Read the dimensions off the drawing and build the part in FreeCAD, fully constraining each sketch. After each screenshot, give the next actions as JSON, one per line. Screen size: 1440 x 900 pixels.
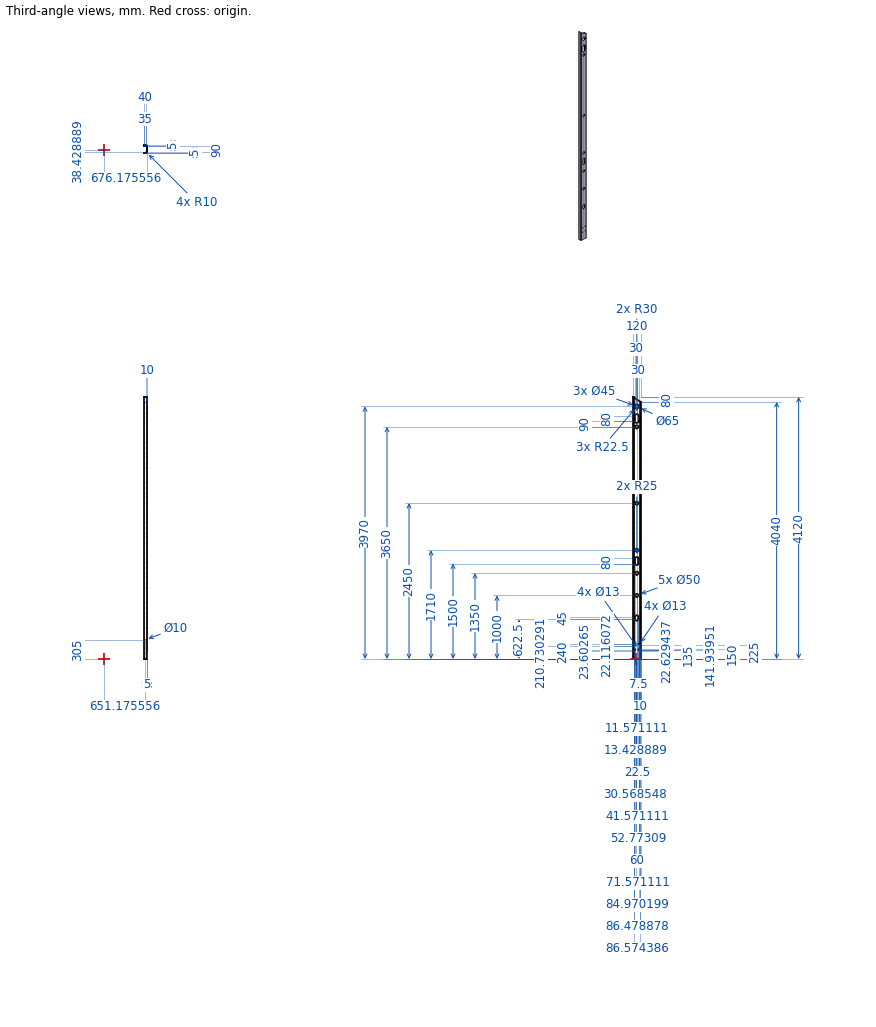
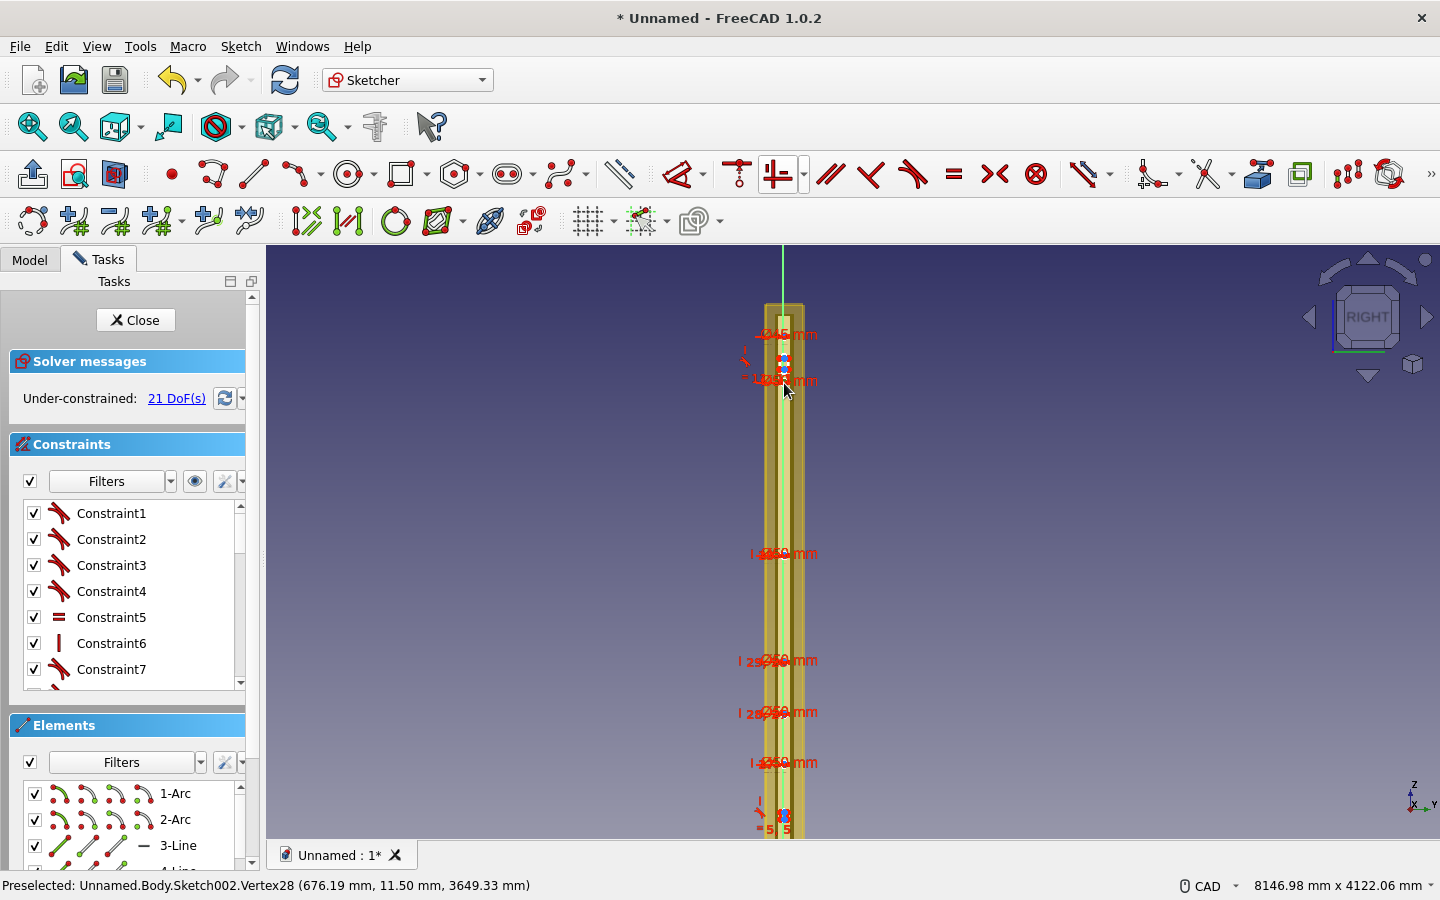
{"action": "left_click", "coordinate": [784, 556]}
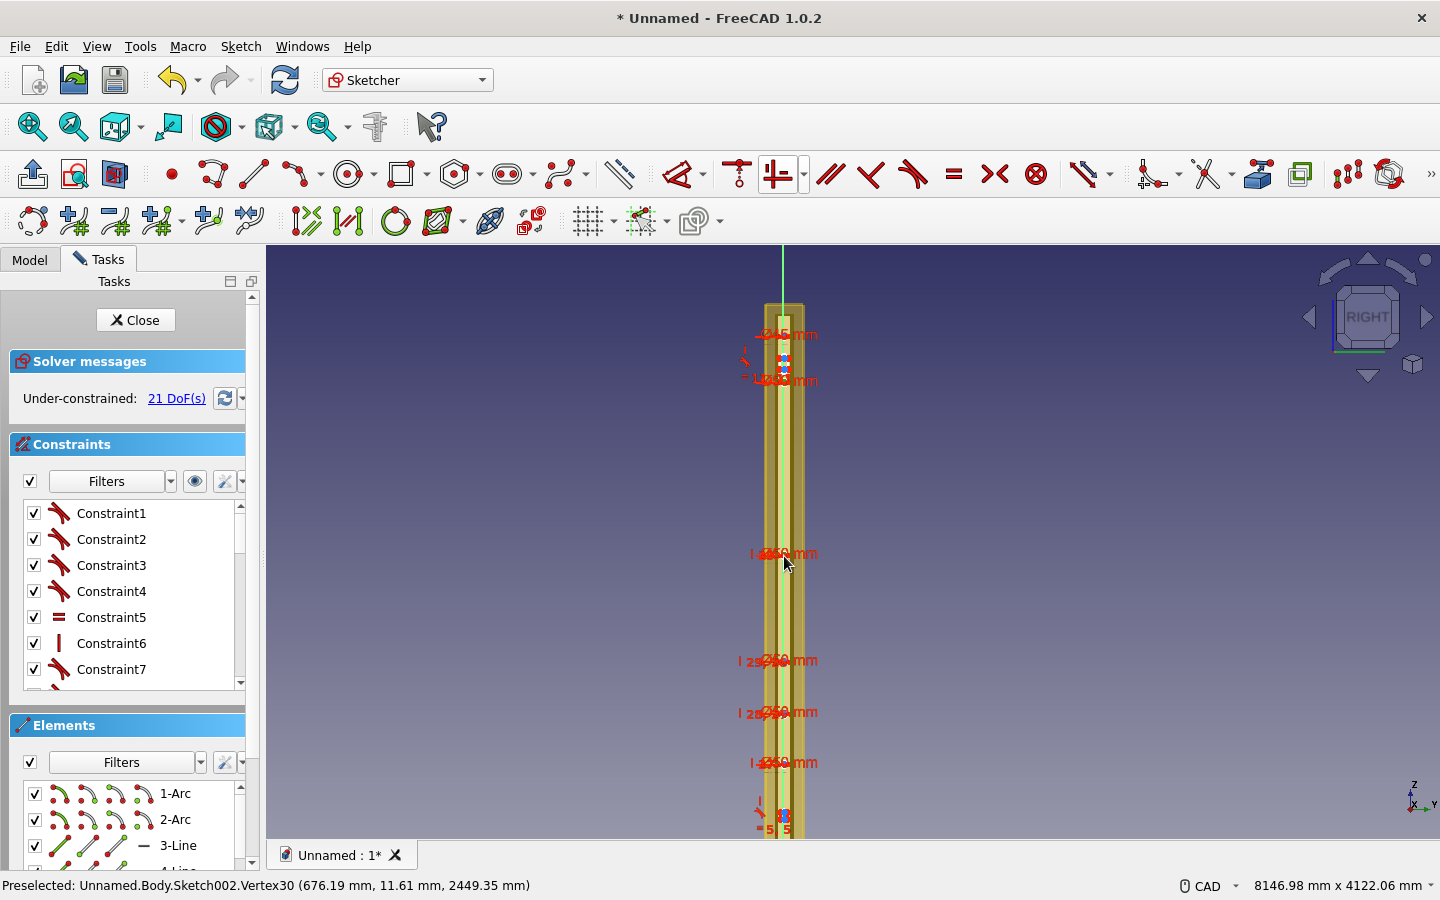
{"action": "key", "text": "v"}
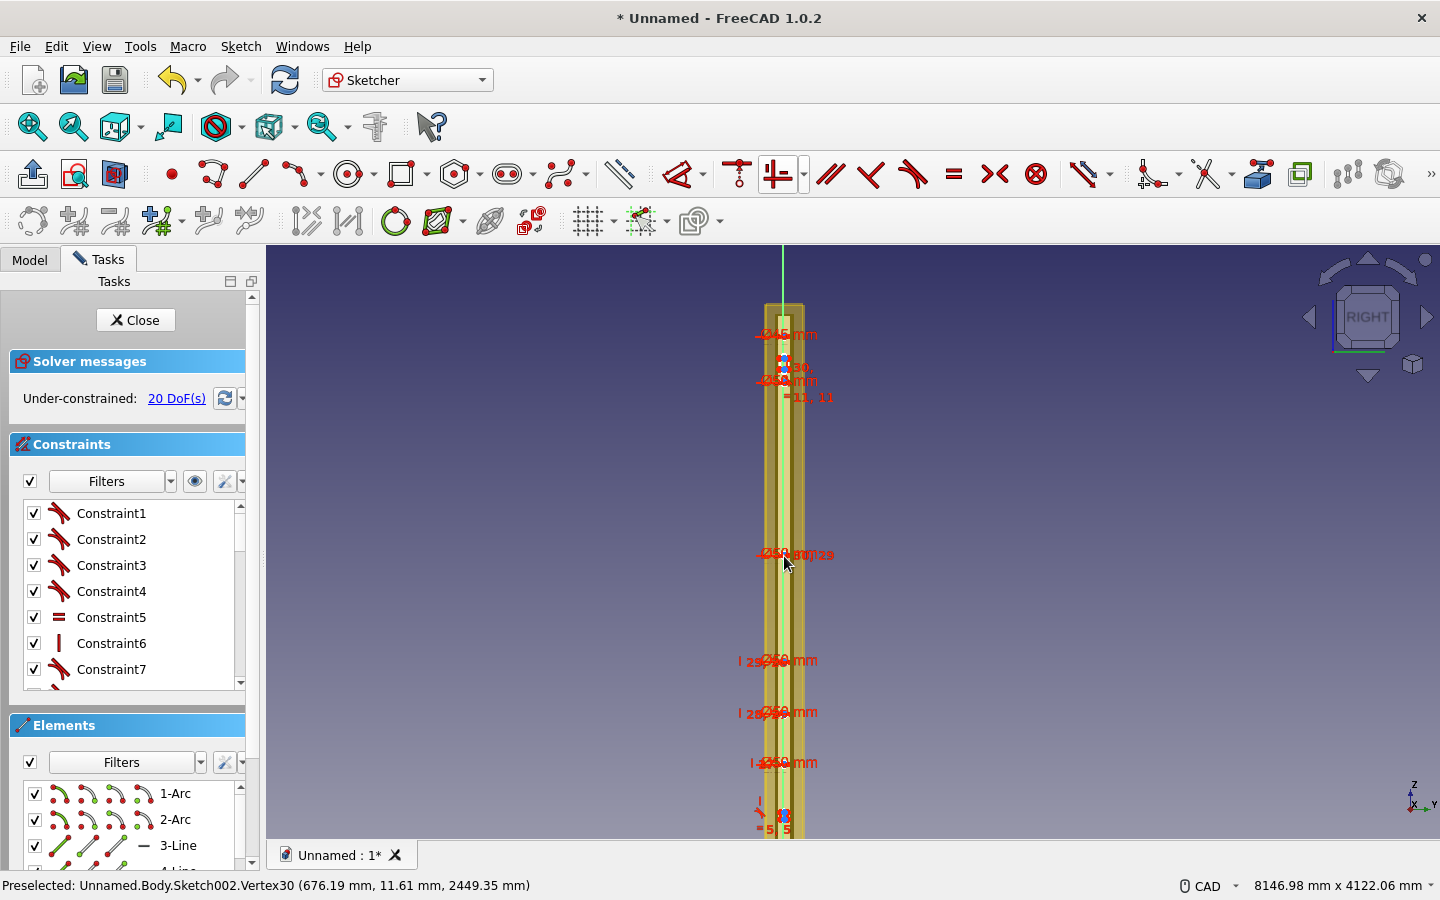
{"action": "key", "text": "d"}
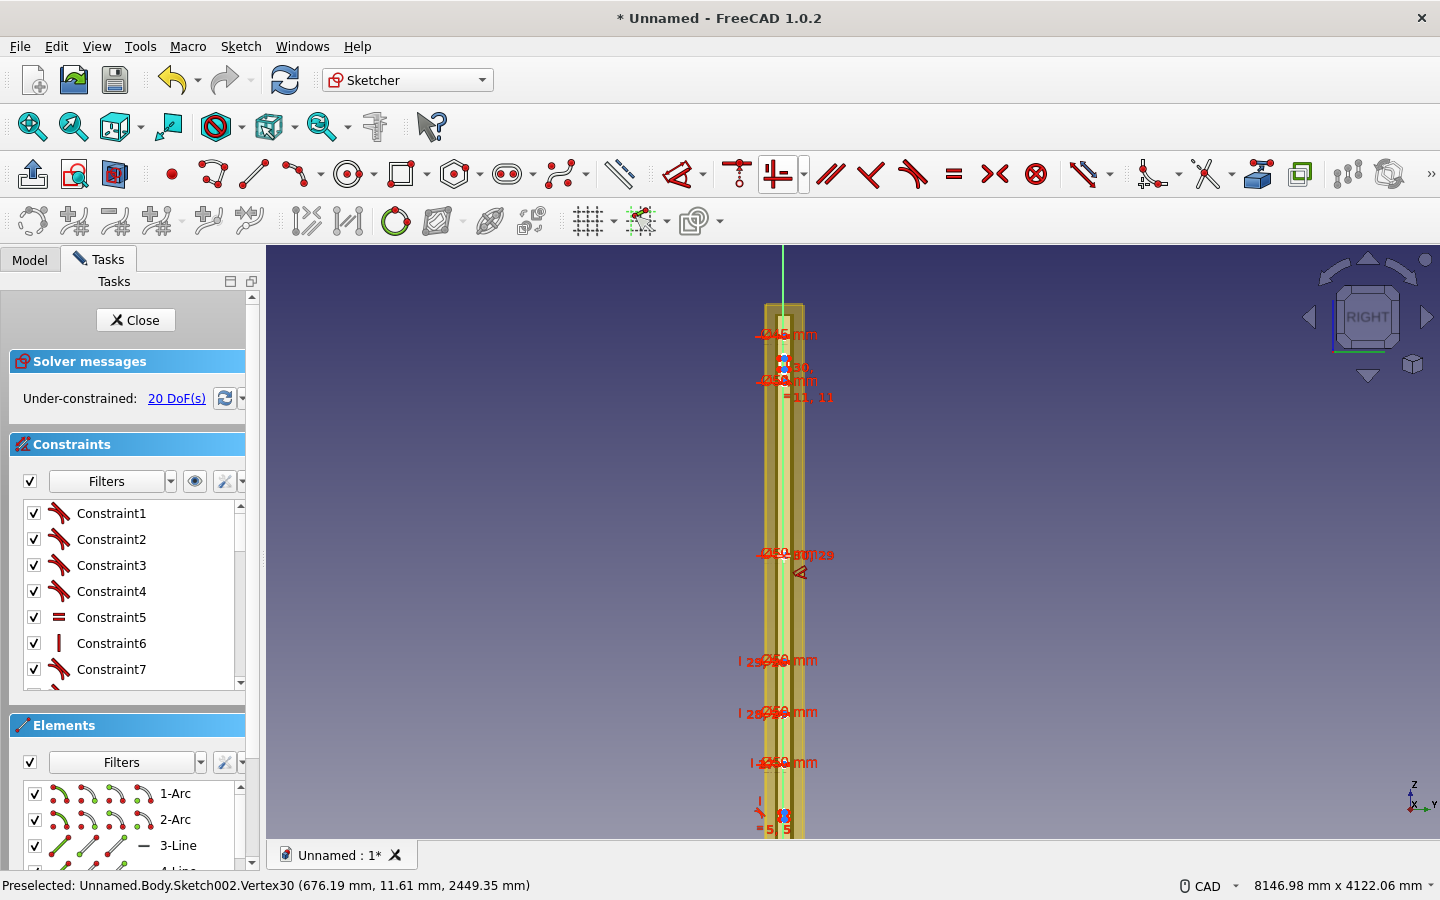
{"action": "scroll", "coordinate": [785, 381], "scroll_direction": "down", "scroll_amount": 2}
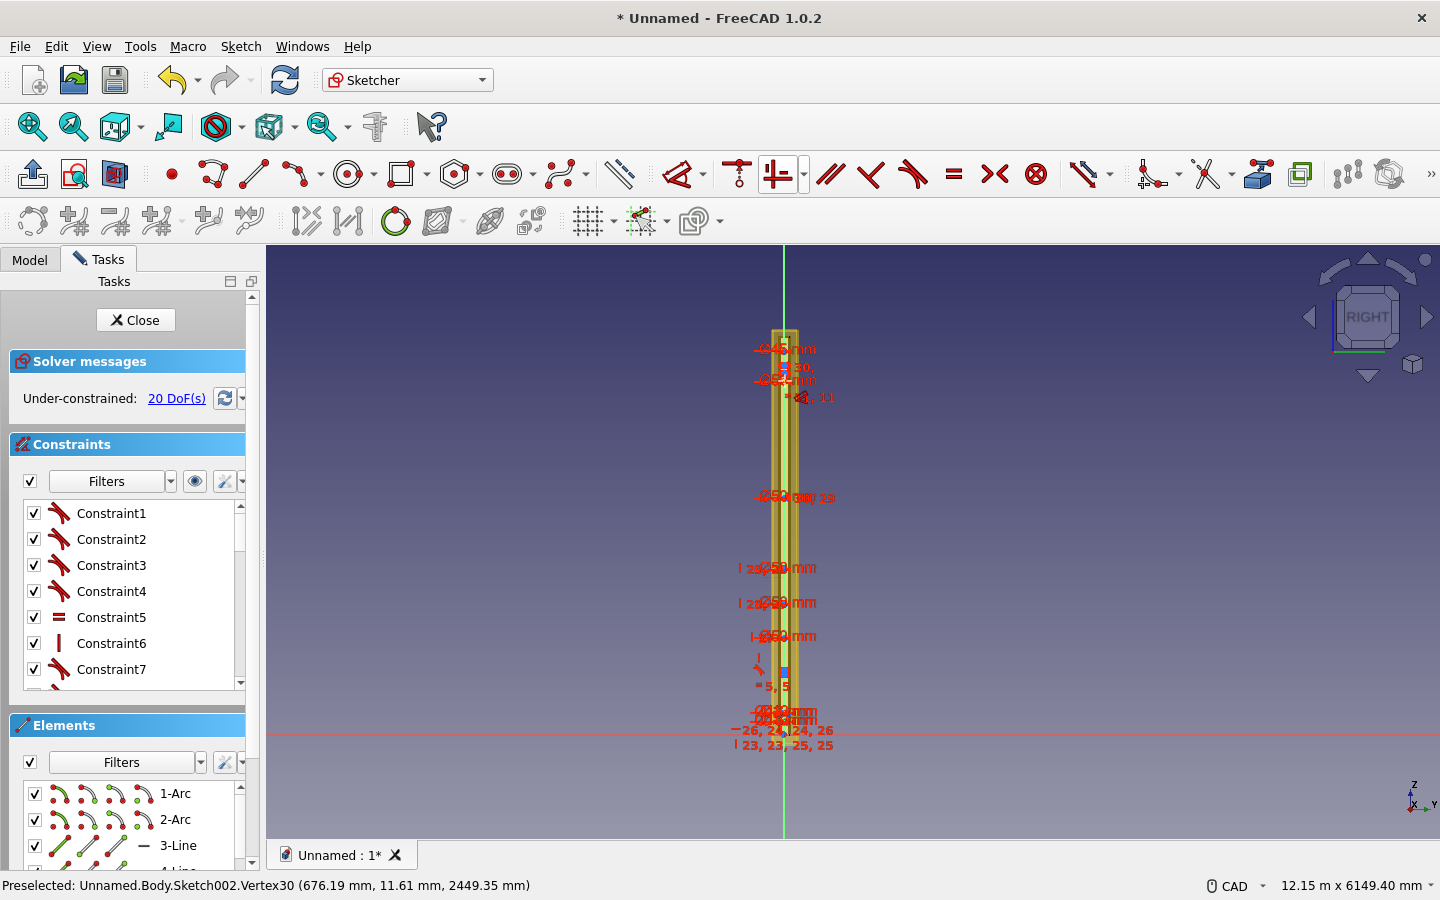
{"action": "scroll", "coordinate": [785, 677], "scroll_direction": "up", "scroll_amount": 15}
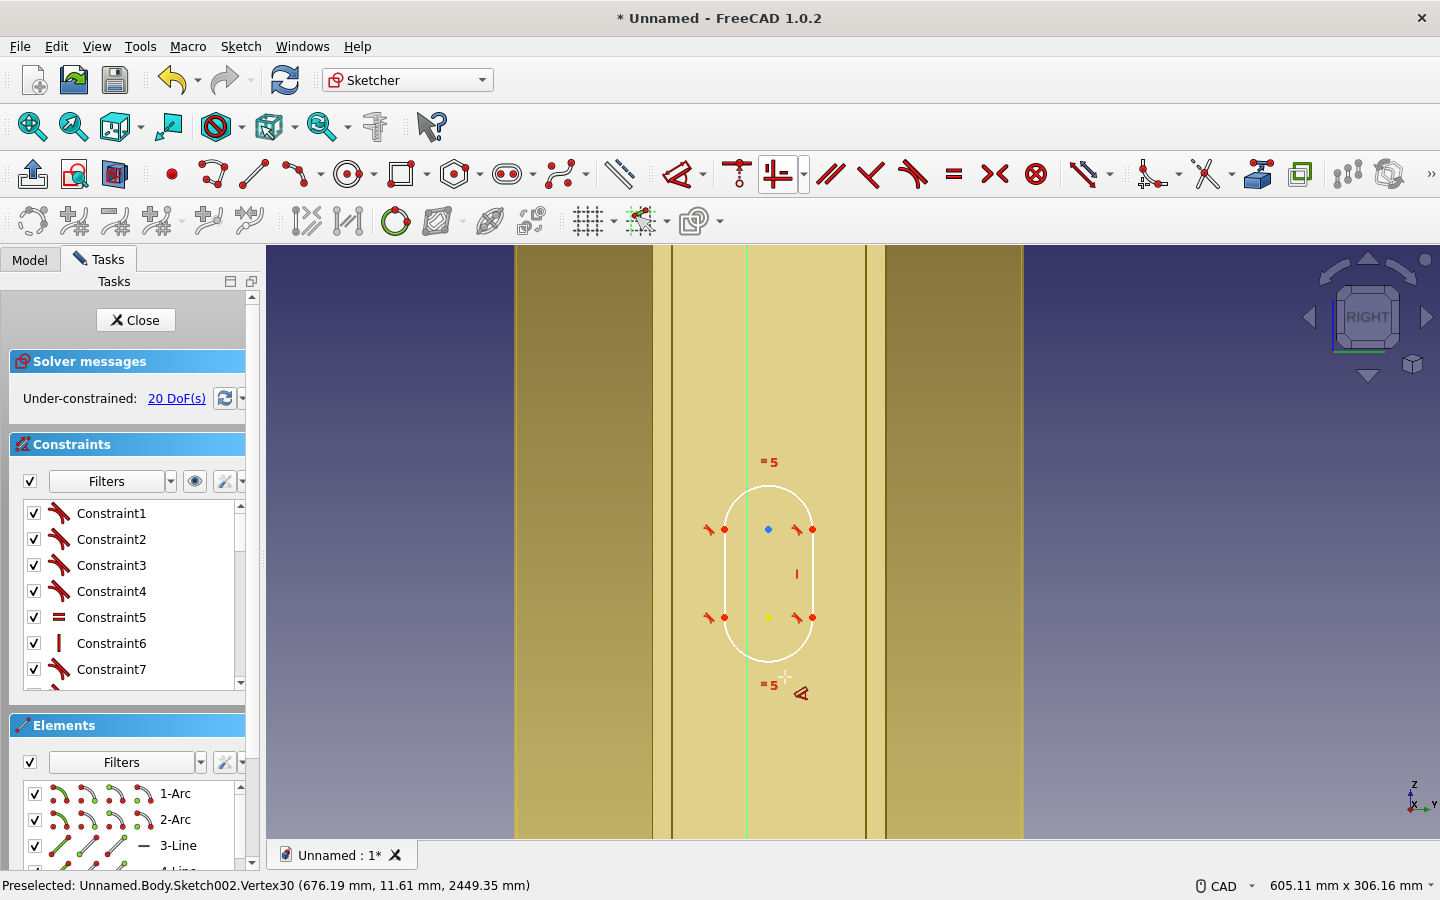
{"action": "left_click", "coordinate": [769, 662]}
{"action": "left_click", "coordinate": [769, 694]}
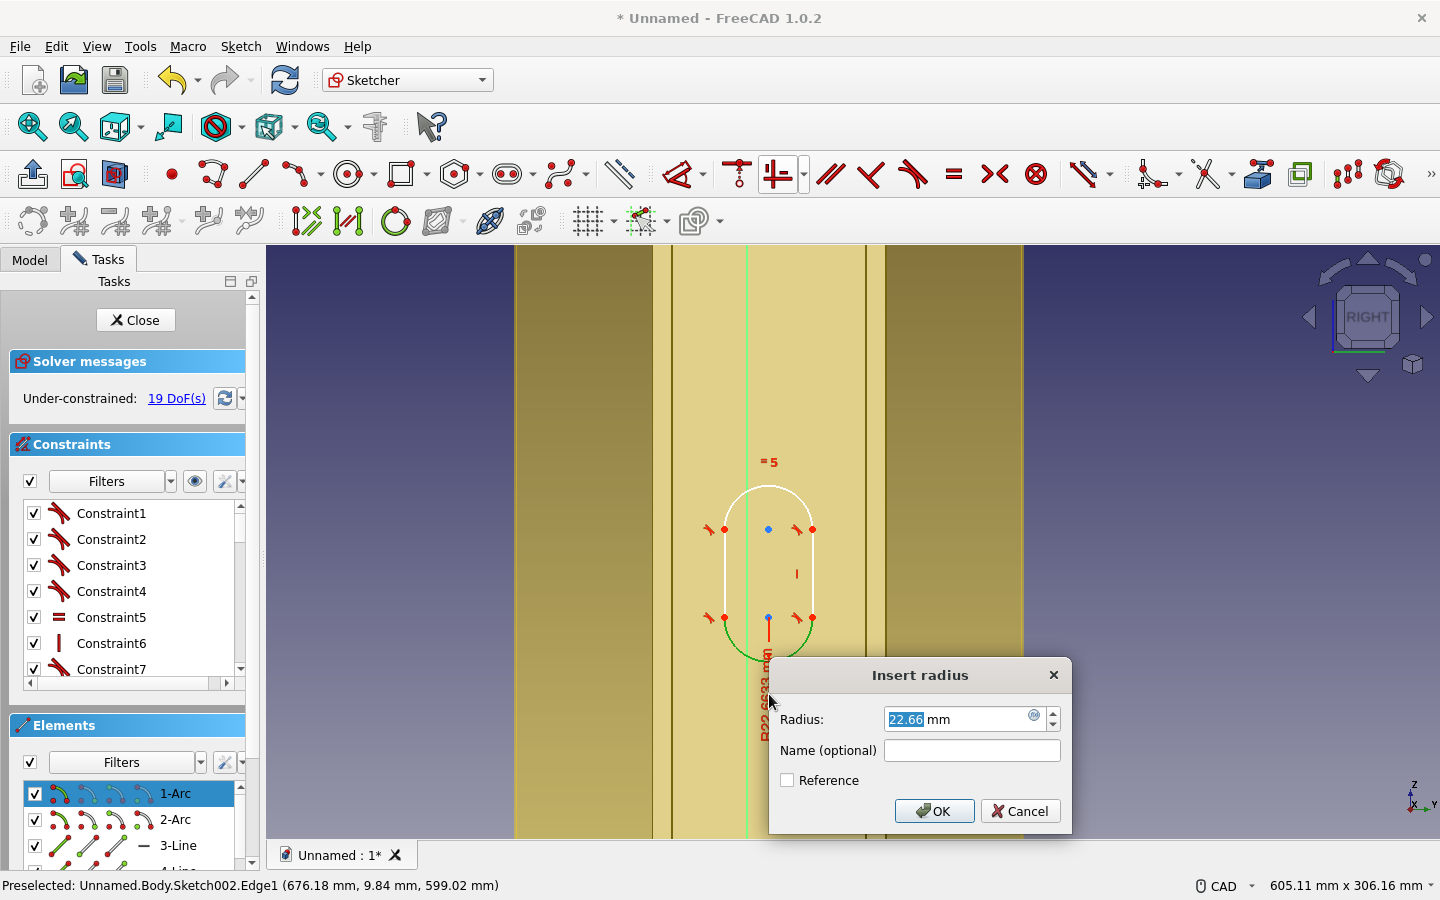
{"action": "type", "text": "22.5"}
{"action": "key", "text": "Return"}